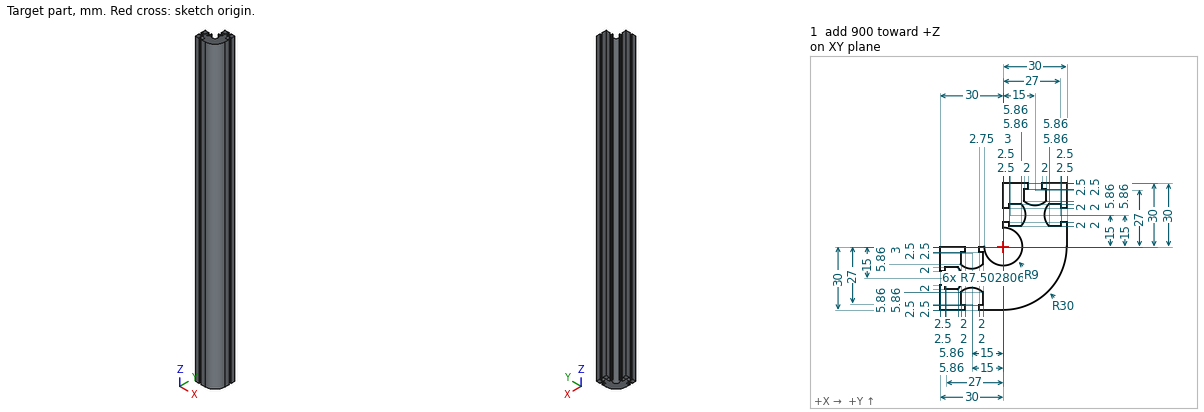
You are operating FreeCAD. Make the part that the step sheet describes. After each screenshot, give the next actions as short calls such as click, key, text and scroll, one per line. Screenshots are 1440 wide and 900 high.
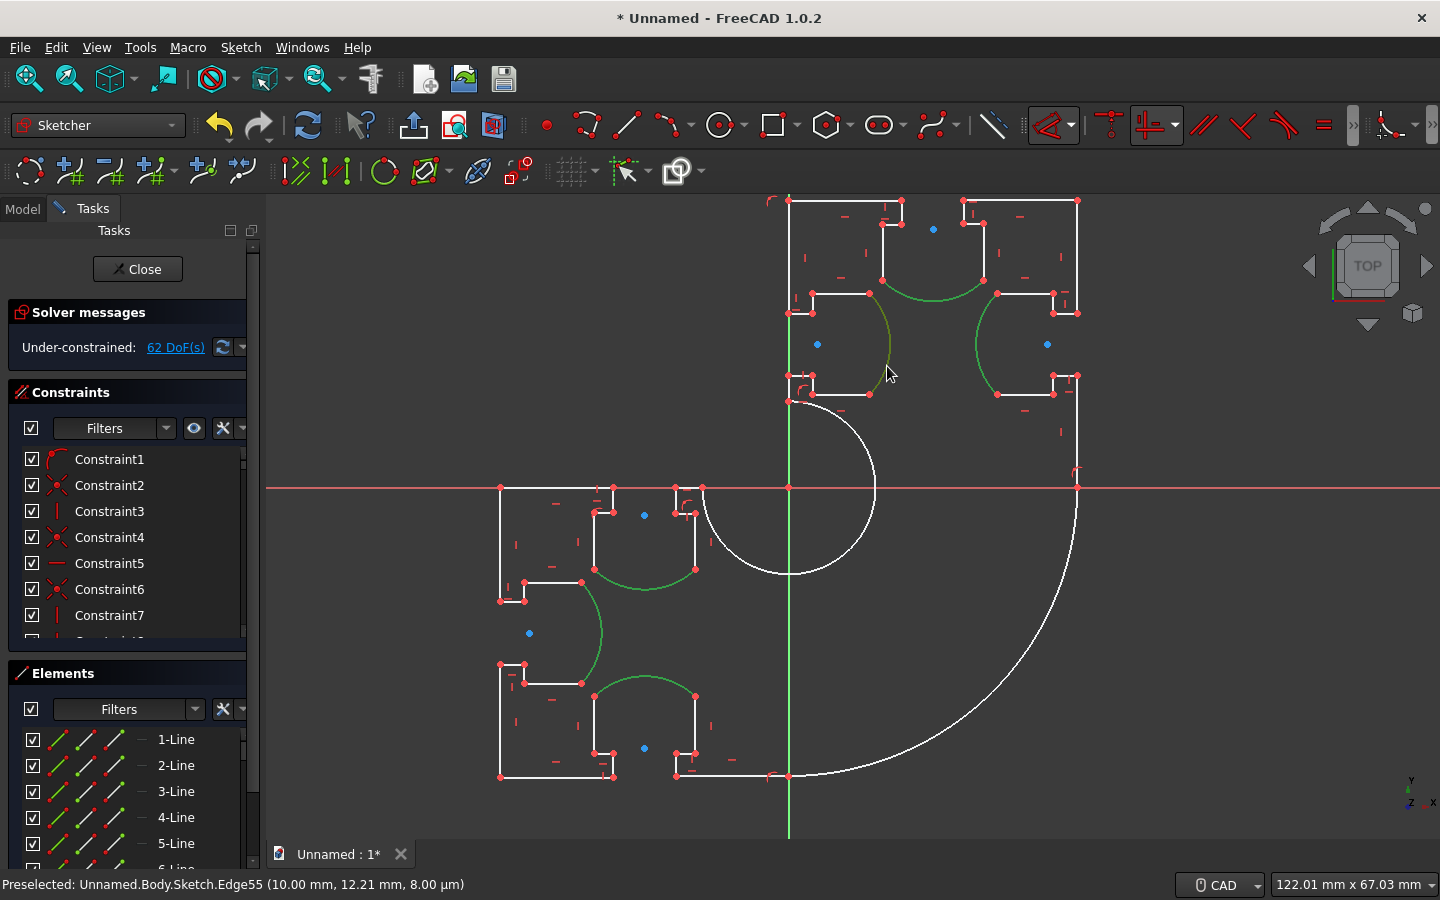
click(1324, 126)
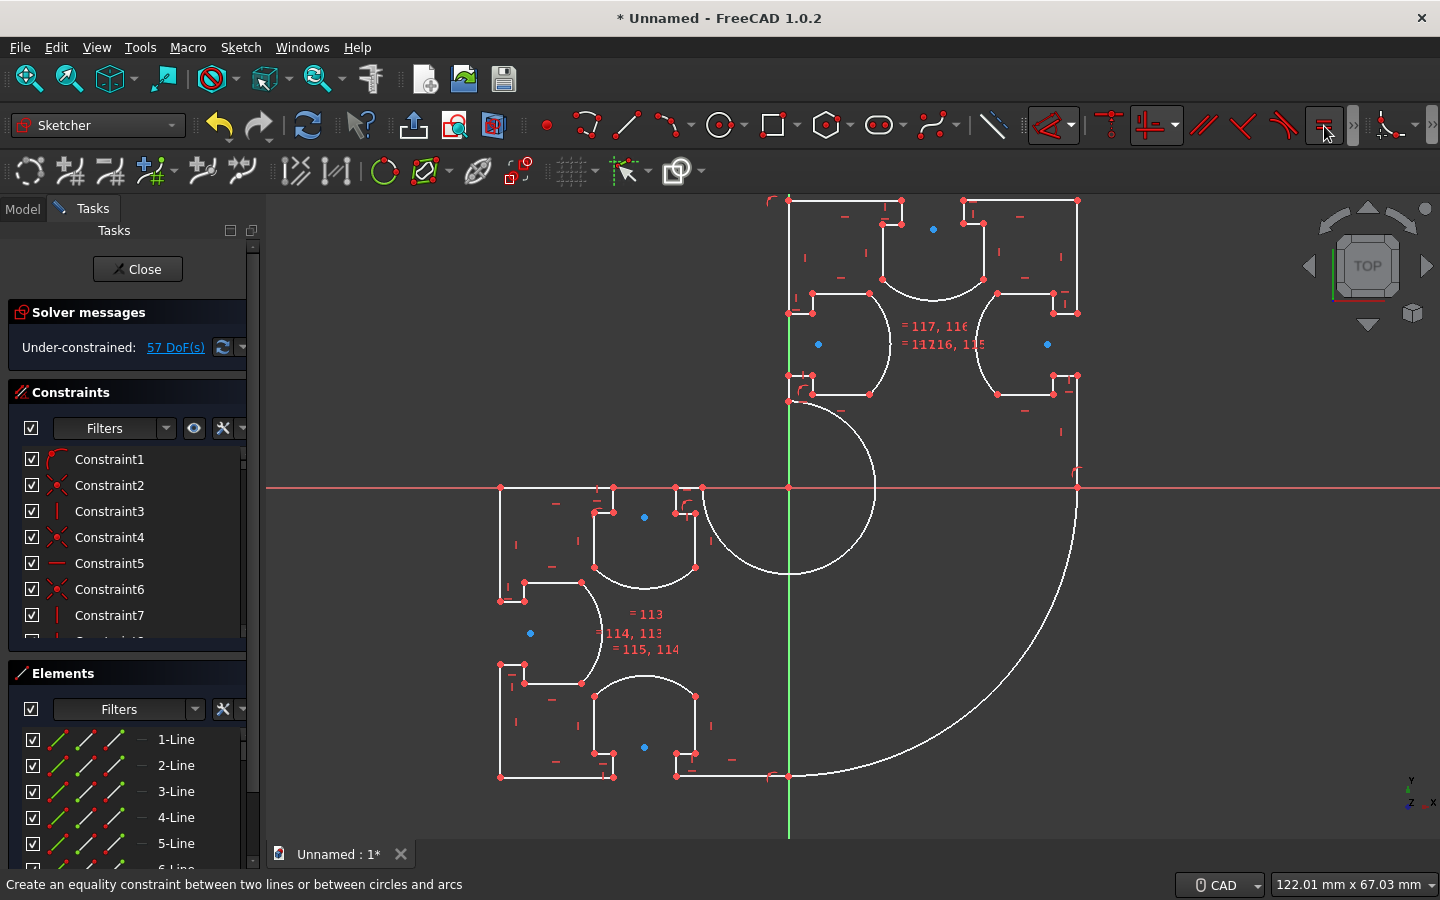
click(1048, 126)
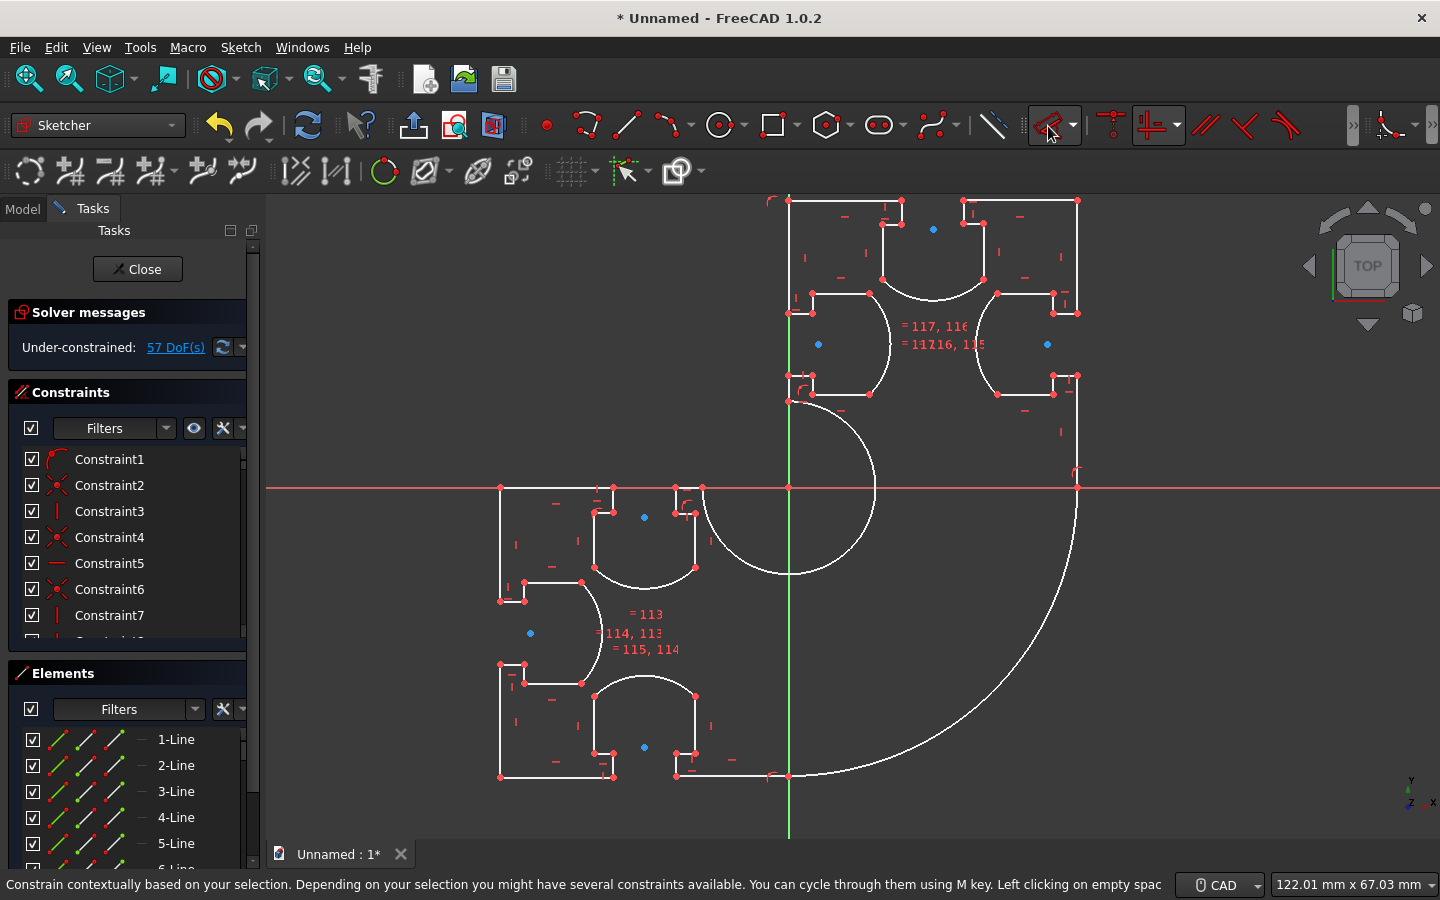
click(623, 585)
click(664, 619)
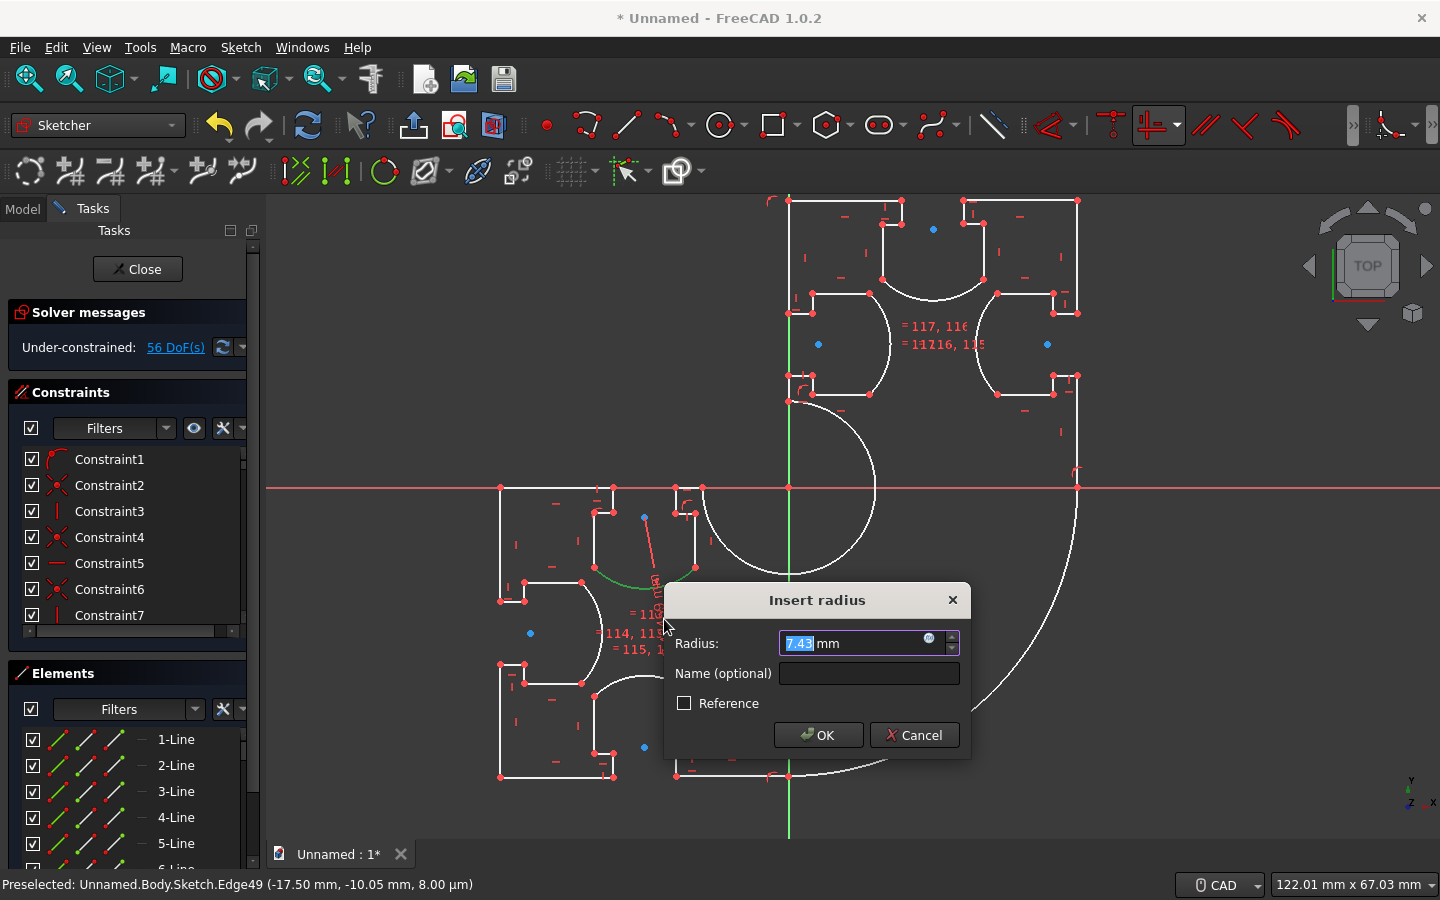
text(7.502806)
key(Return)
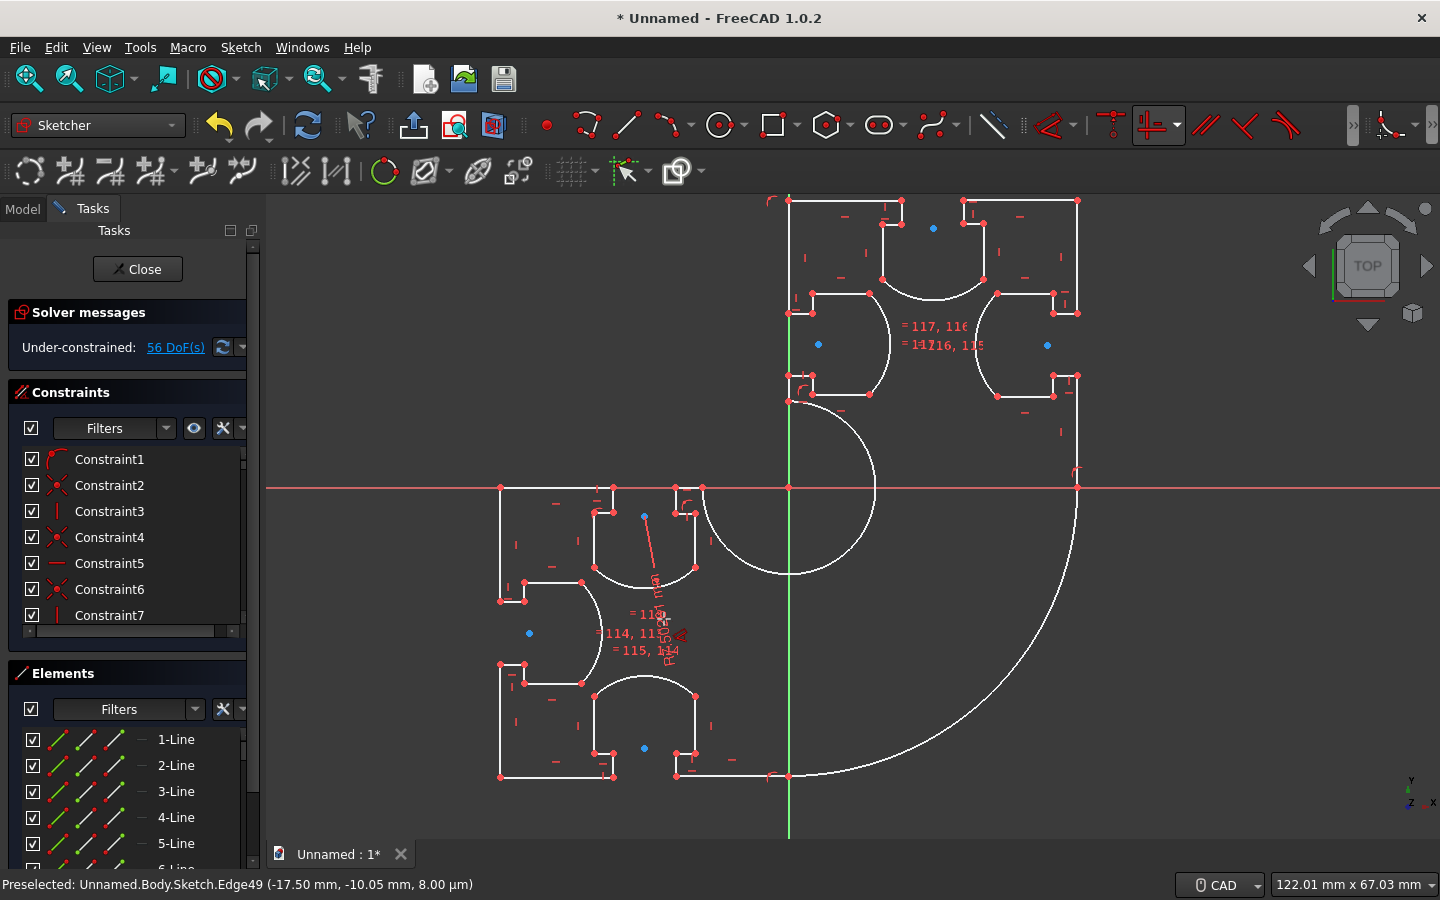
click(920, 745)
click(935, 774)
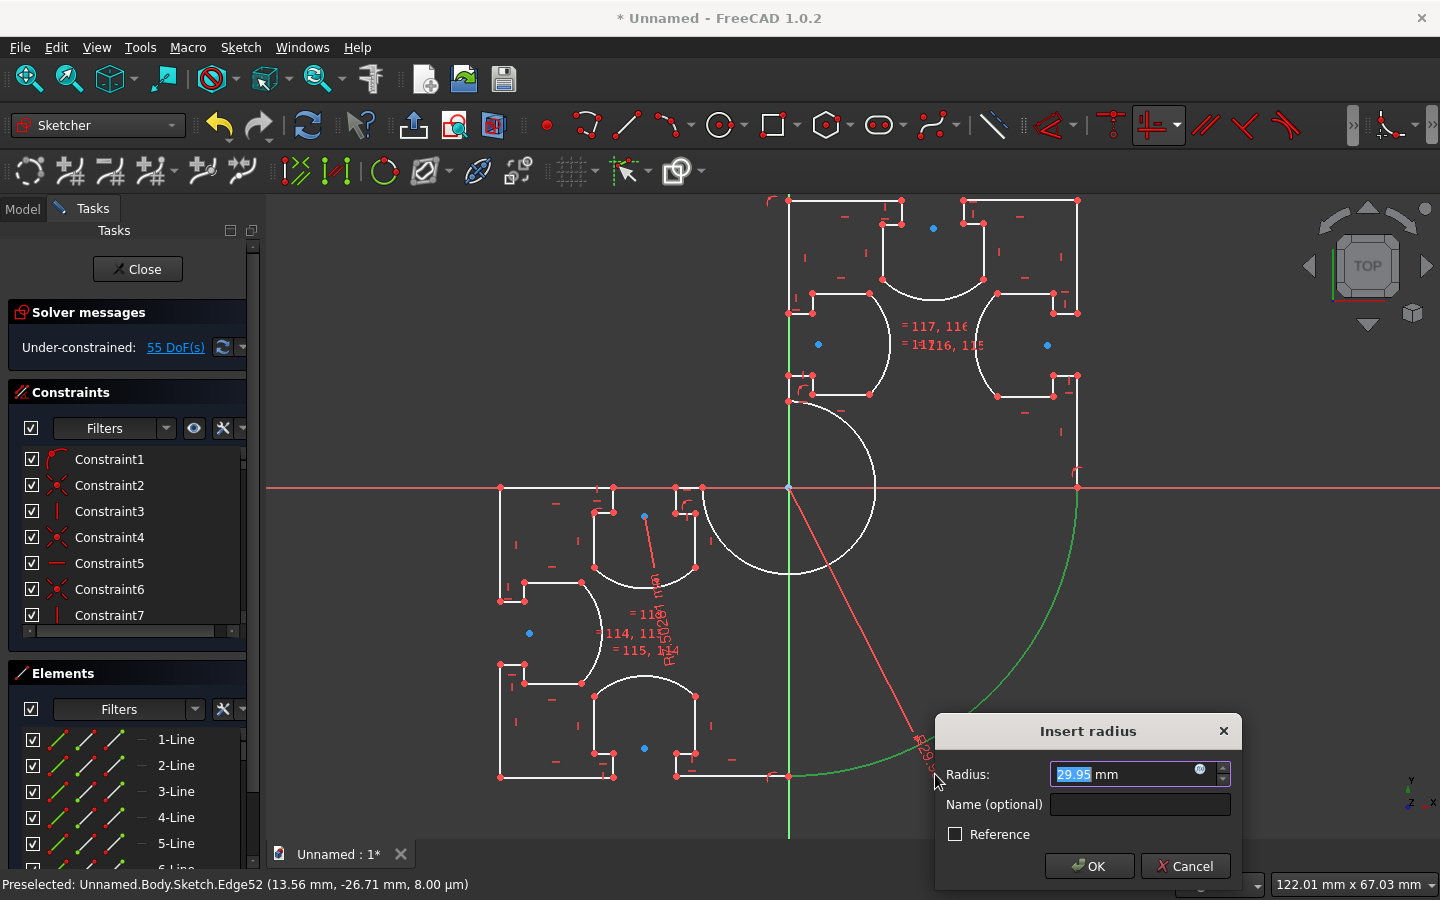
text(30)
key(Return)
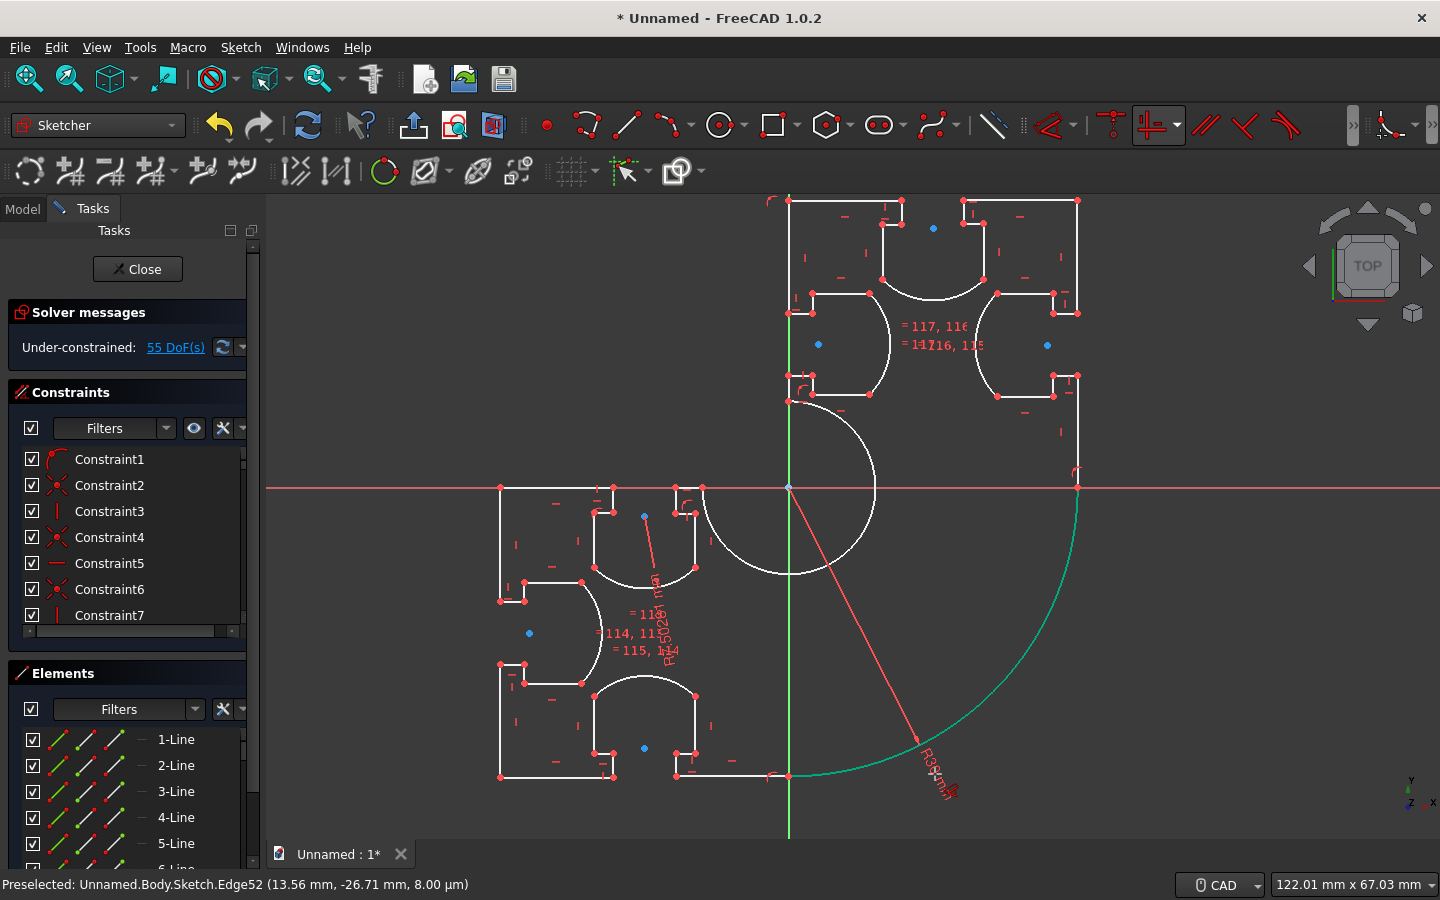
click(775, 573)
click(770, 605)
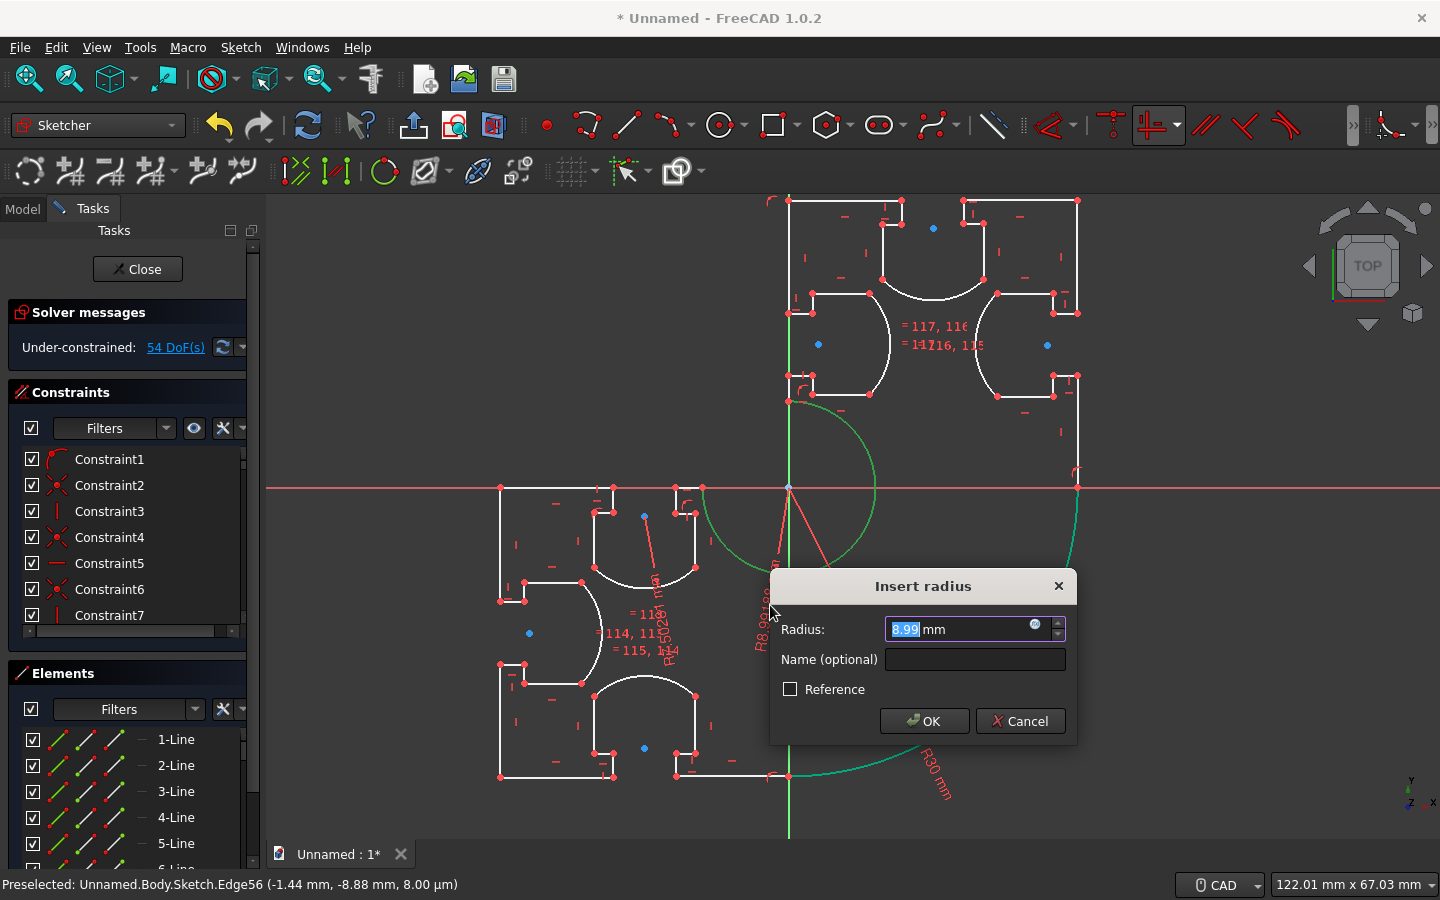
text(9)
key(Return)